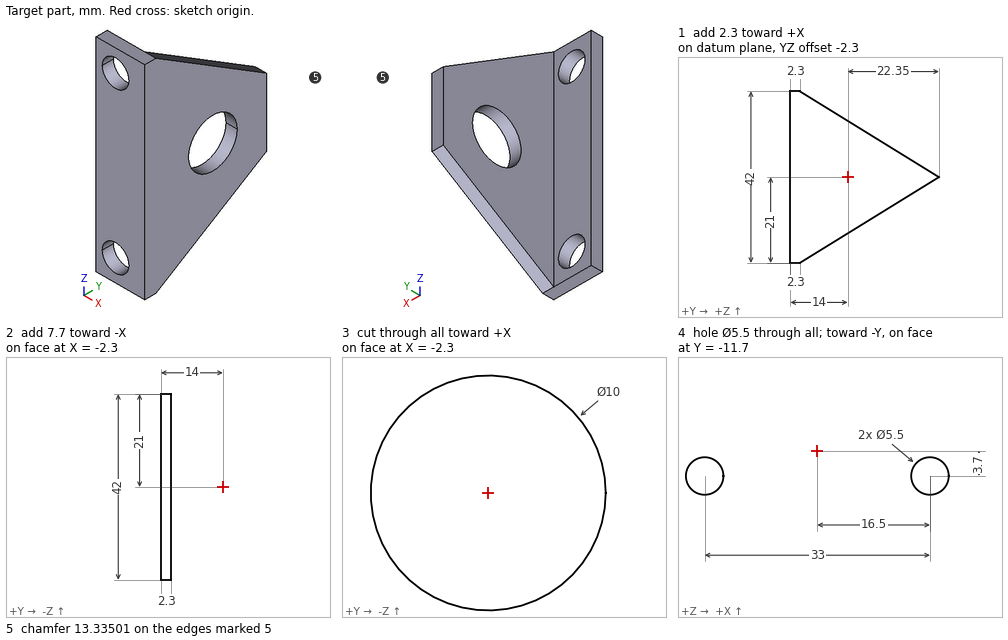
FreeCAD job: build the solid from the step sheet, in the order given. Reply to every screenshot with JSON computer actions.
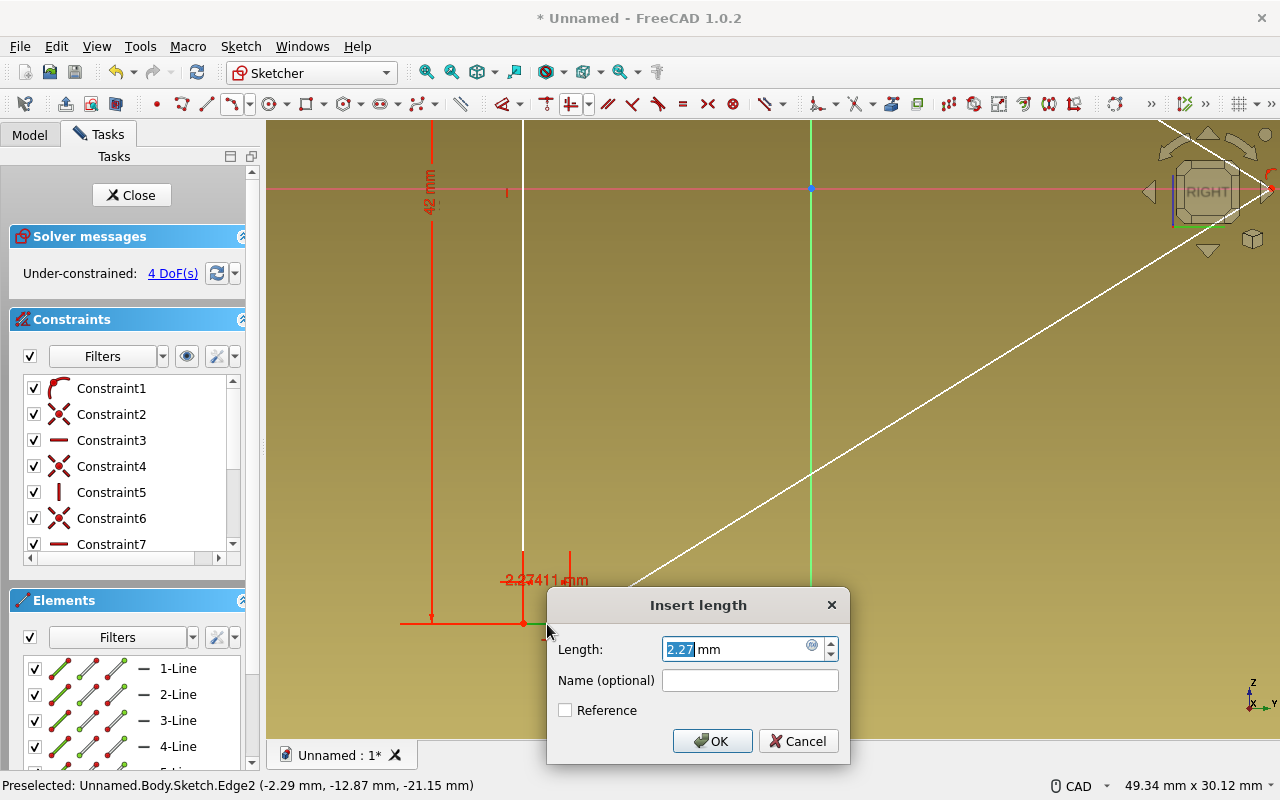
{"action": "type", "text": "2.3"}
{"action": "key", "text": "Return"}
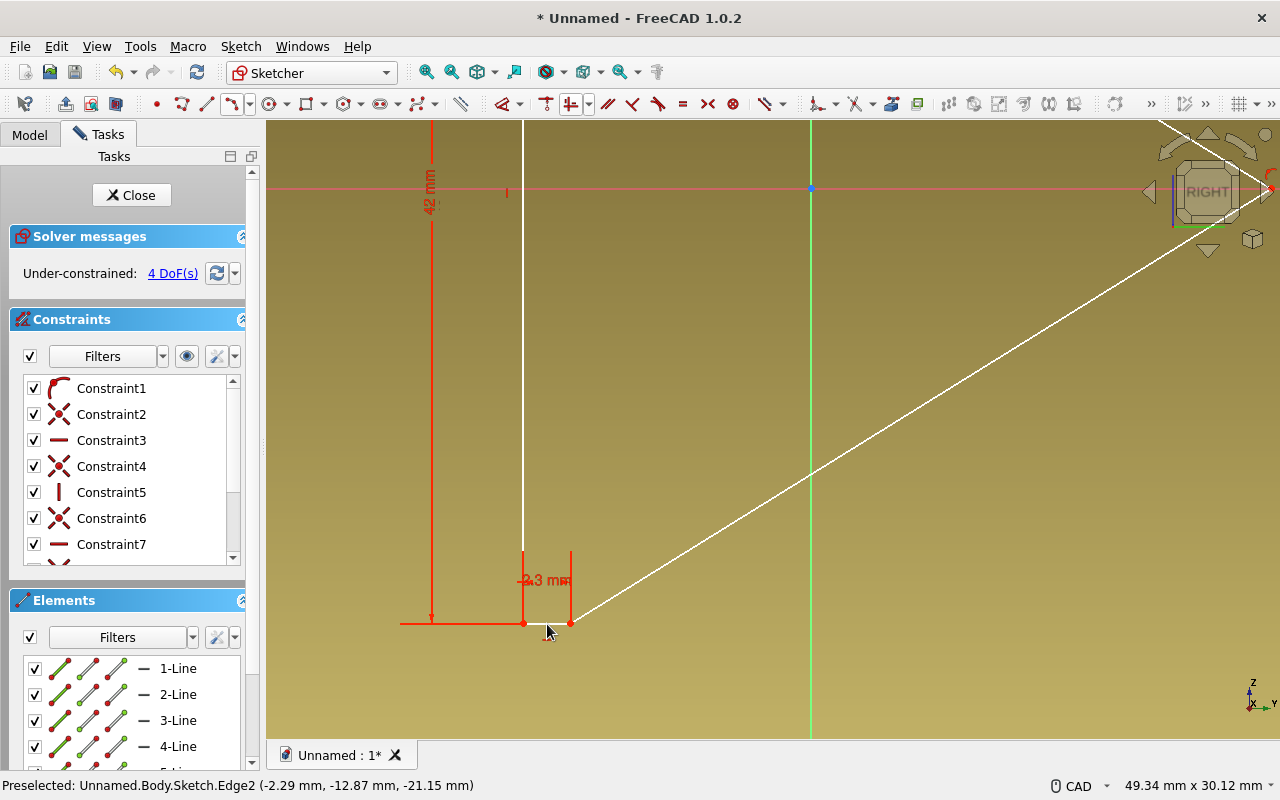
{"action": "scroll", "coordinate": [547, 626], "scroll_direction": "down", "scroll_amount": 4}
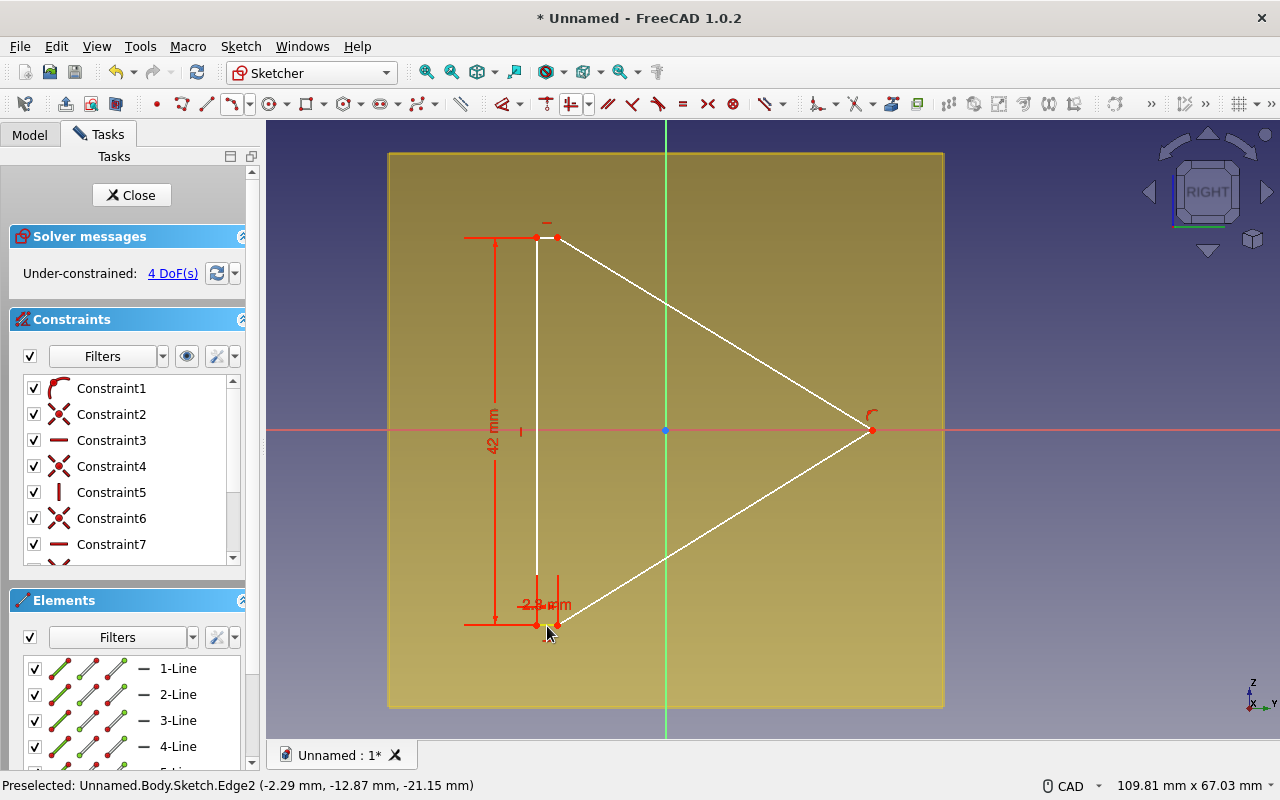
{"action": "scroll", "coordinate": [543, 238], "scroll_direction": "up", "scroll_amount": 4}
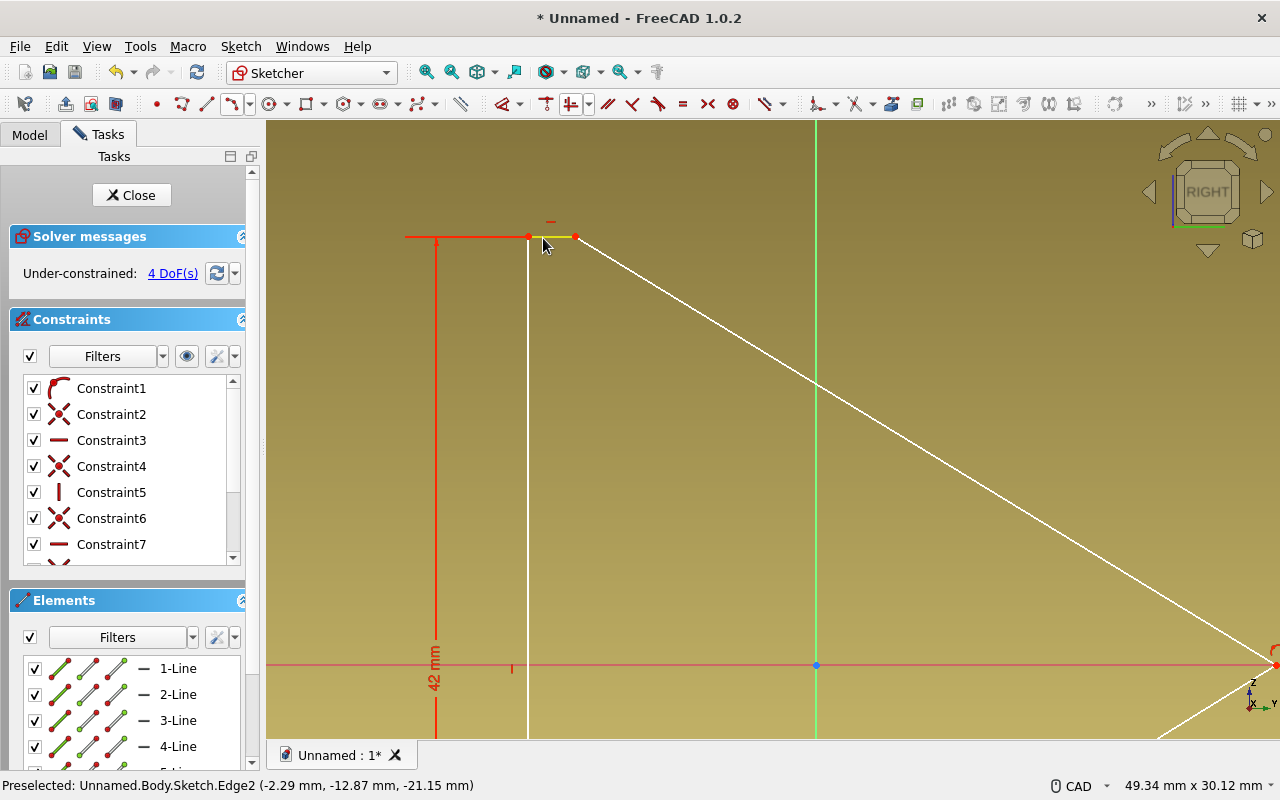
{"action": "left_click", "coordinate": [542, 237]}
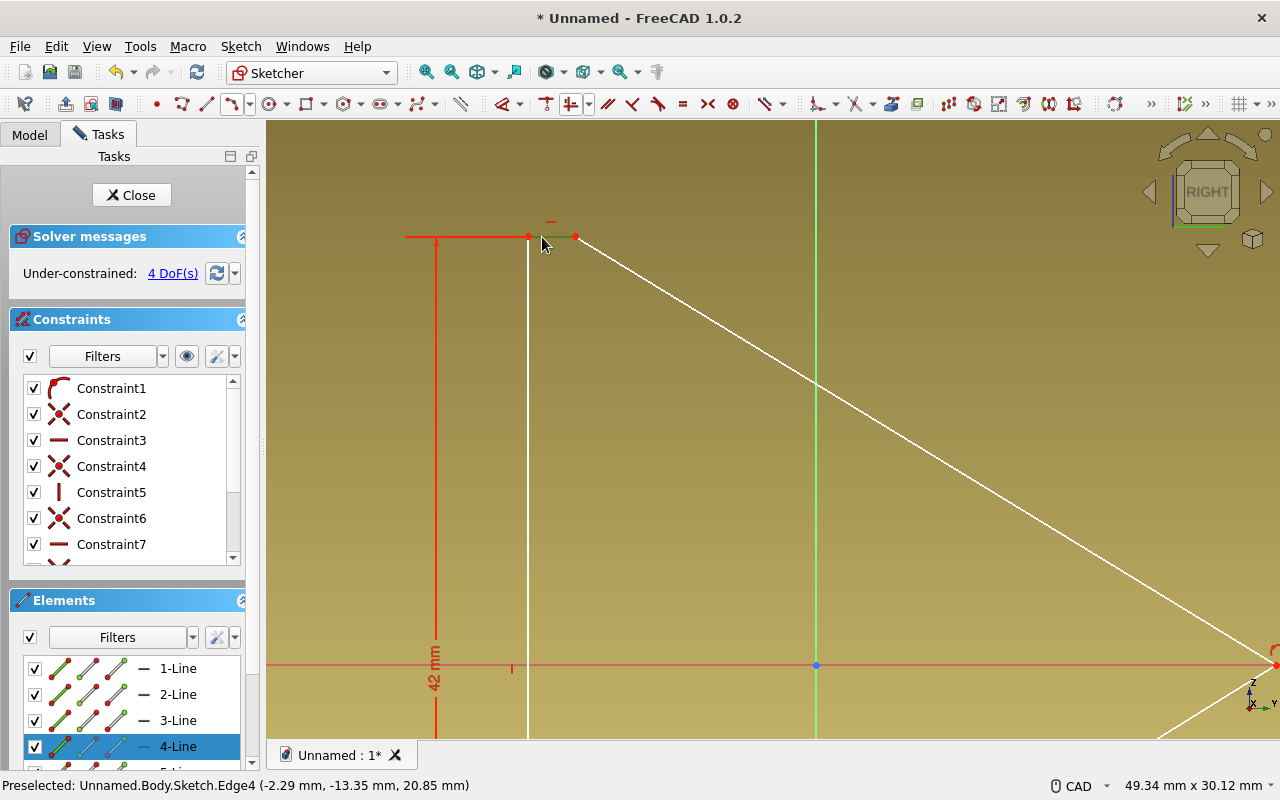
{"action": "key", "text": "l"}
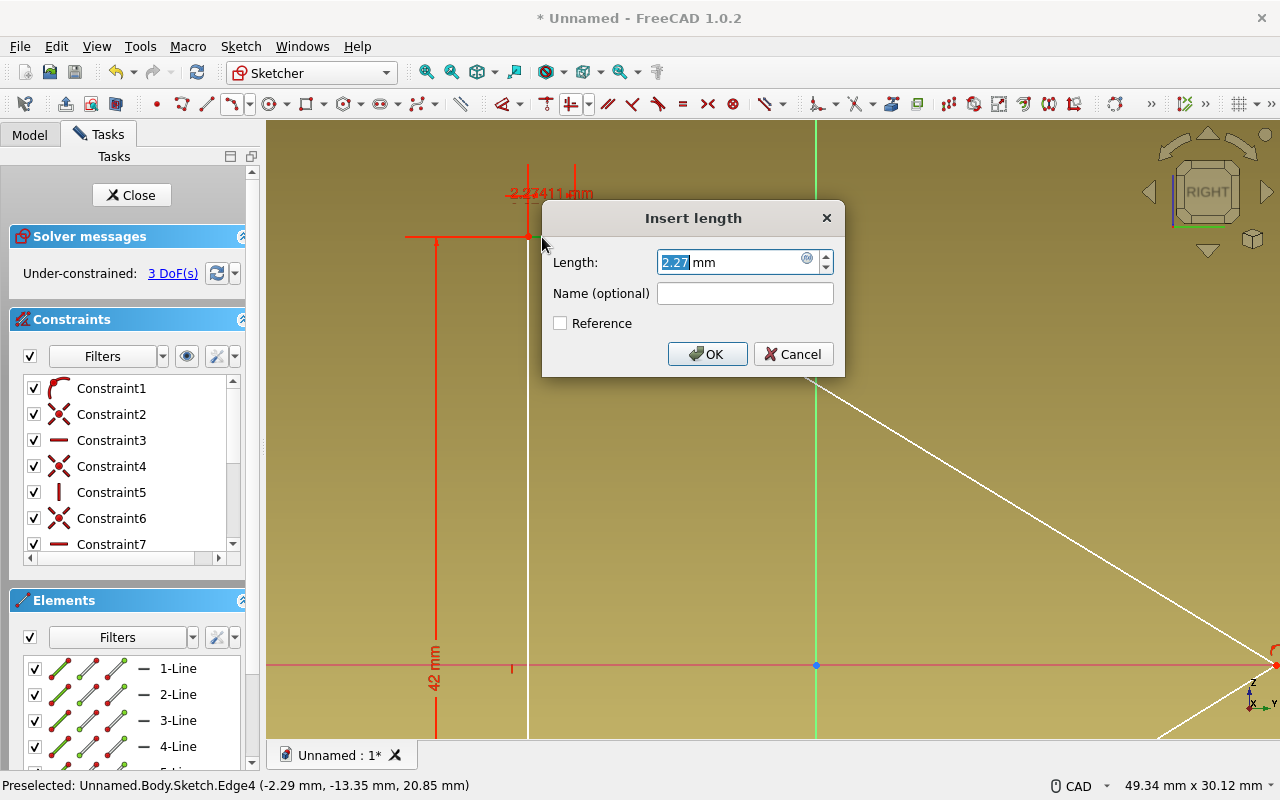
{"action": "type", "text": "2.3"}
{"action": "key", "text": "Return"}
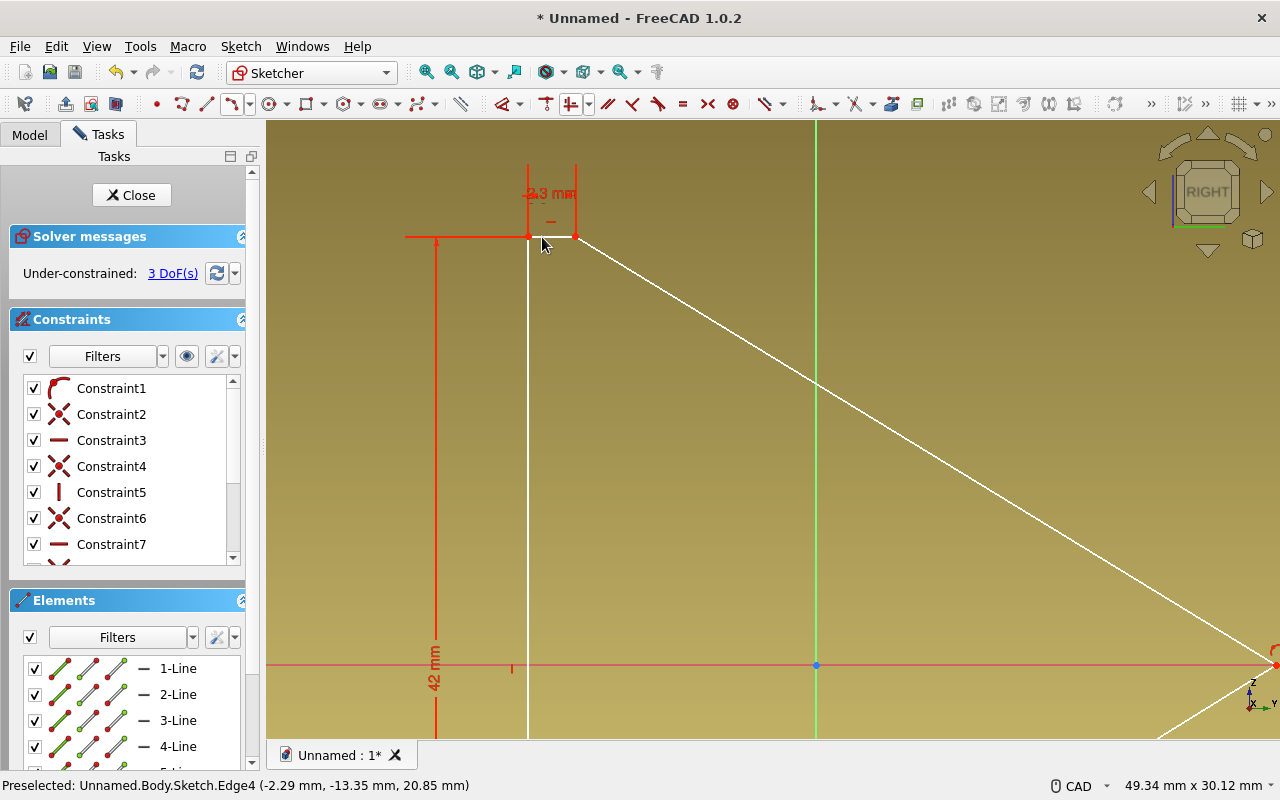
{"action": "scroll", "coordinate": [543, 237], "scroll_direction": "down", "scroll_amount": 4}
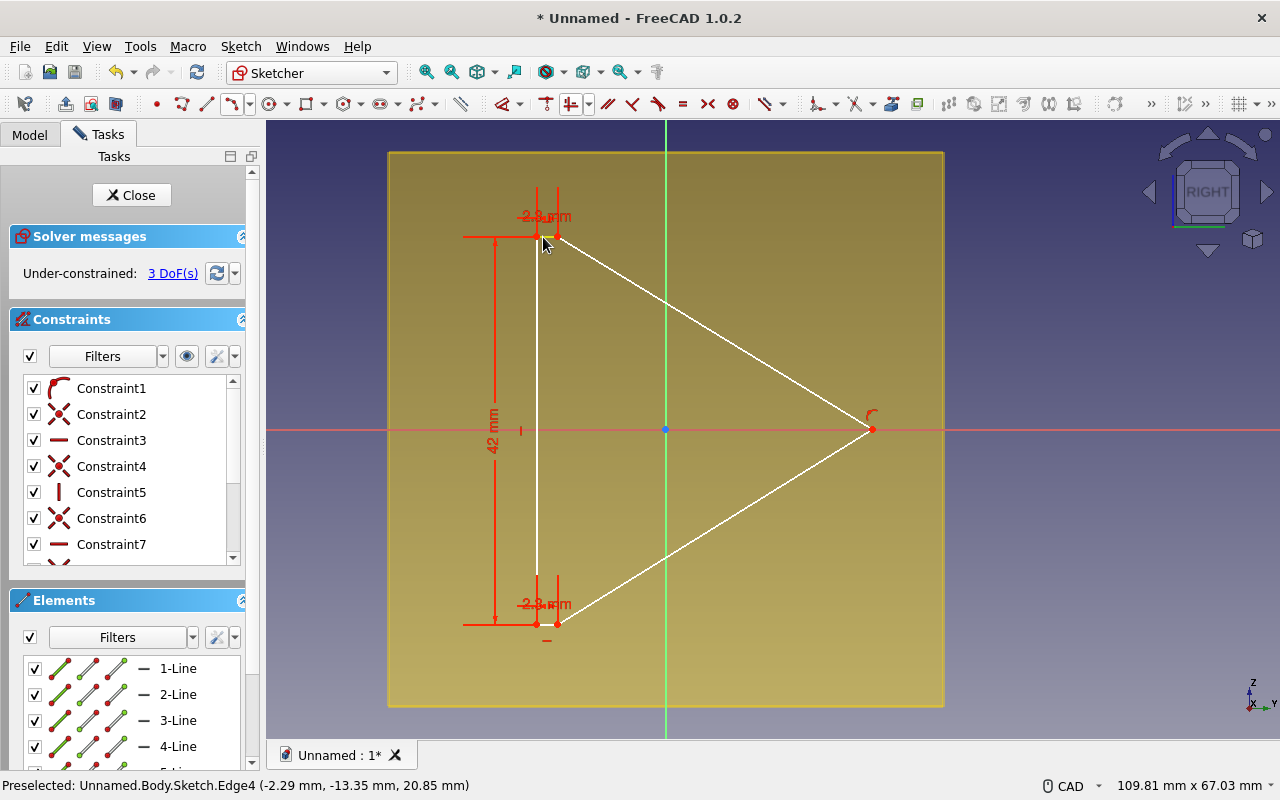
{"action": "left_click", "coordinate": [558, 625]}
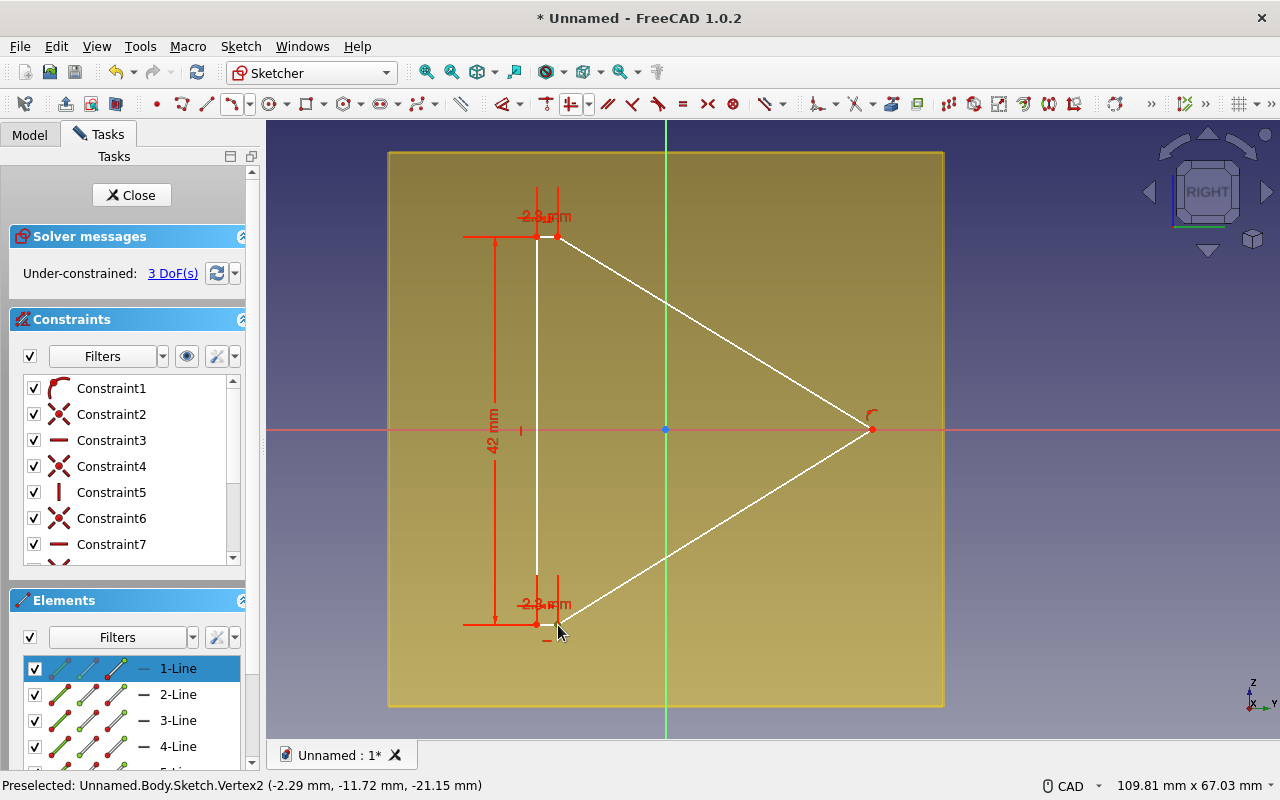
{"action": "key", "text": "i"}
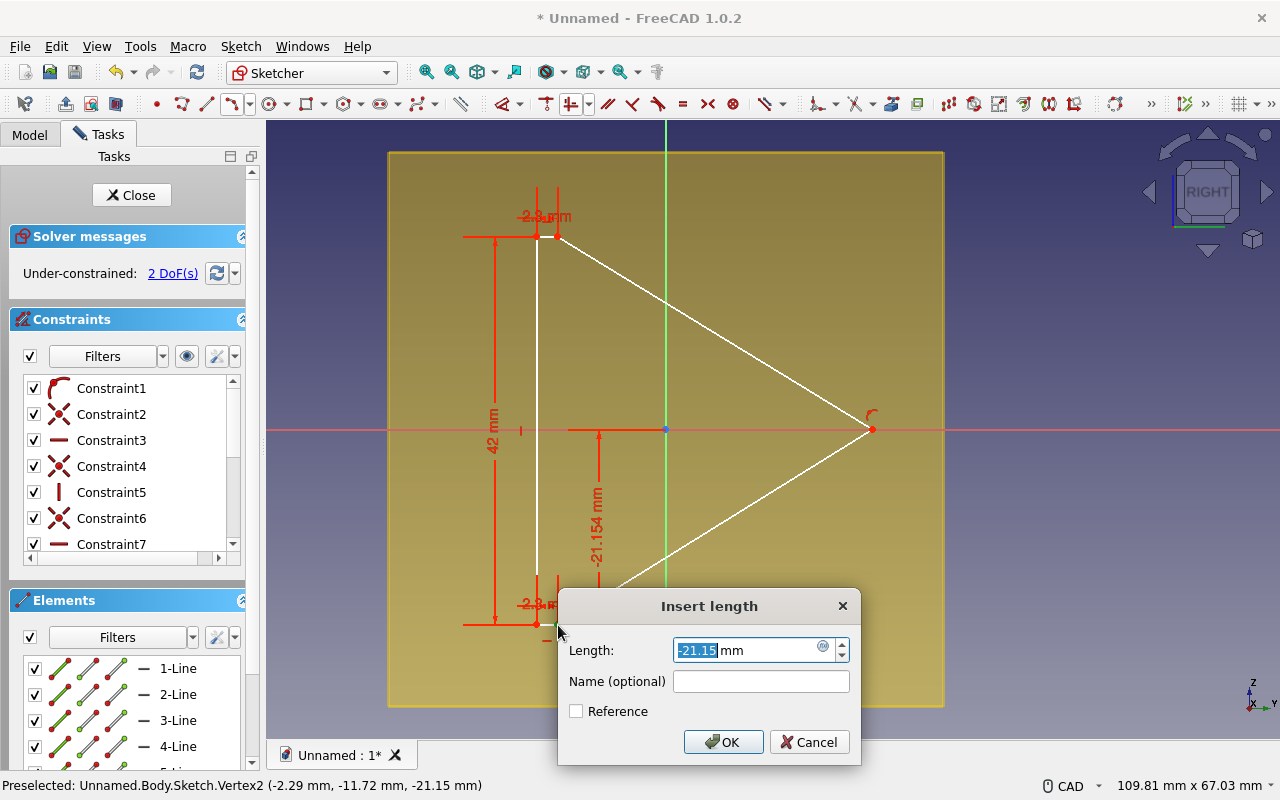
{"action": "type", "text": "-21"}
{"action": "key", "text": "Return"}